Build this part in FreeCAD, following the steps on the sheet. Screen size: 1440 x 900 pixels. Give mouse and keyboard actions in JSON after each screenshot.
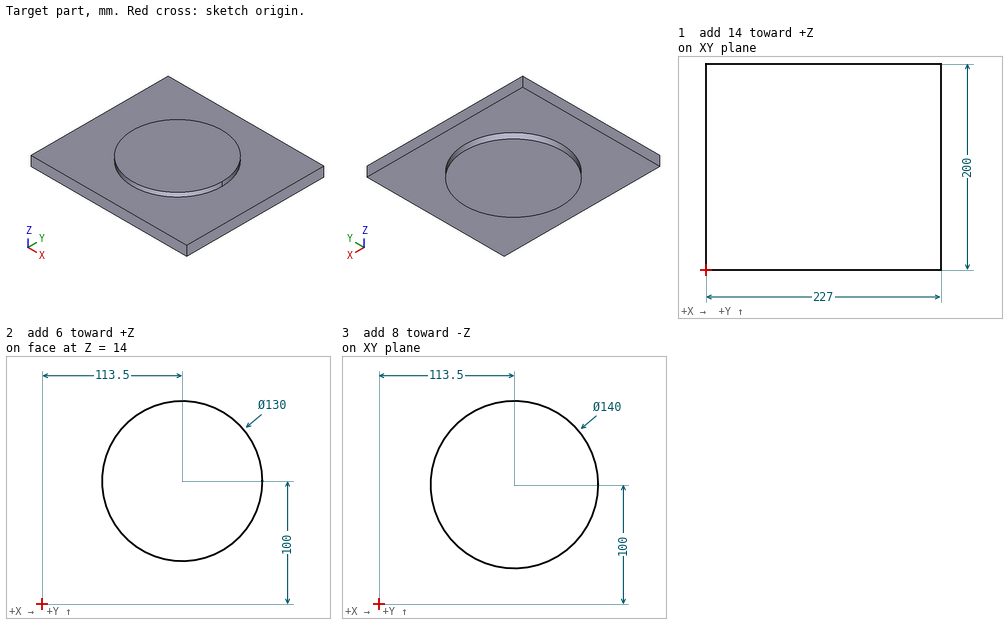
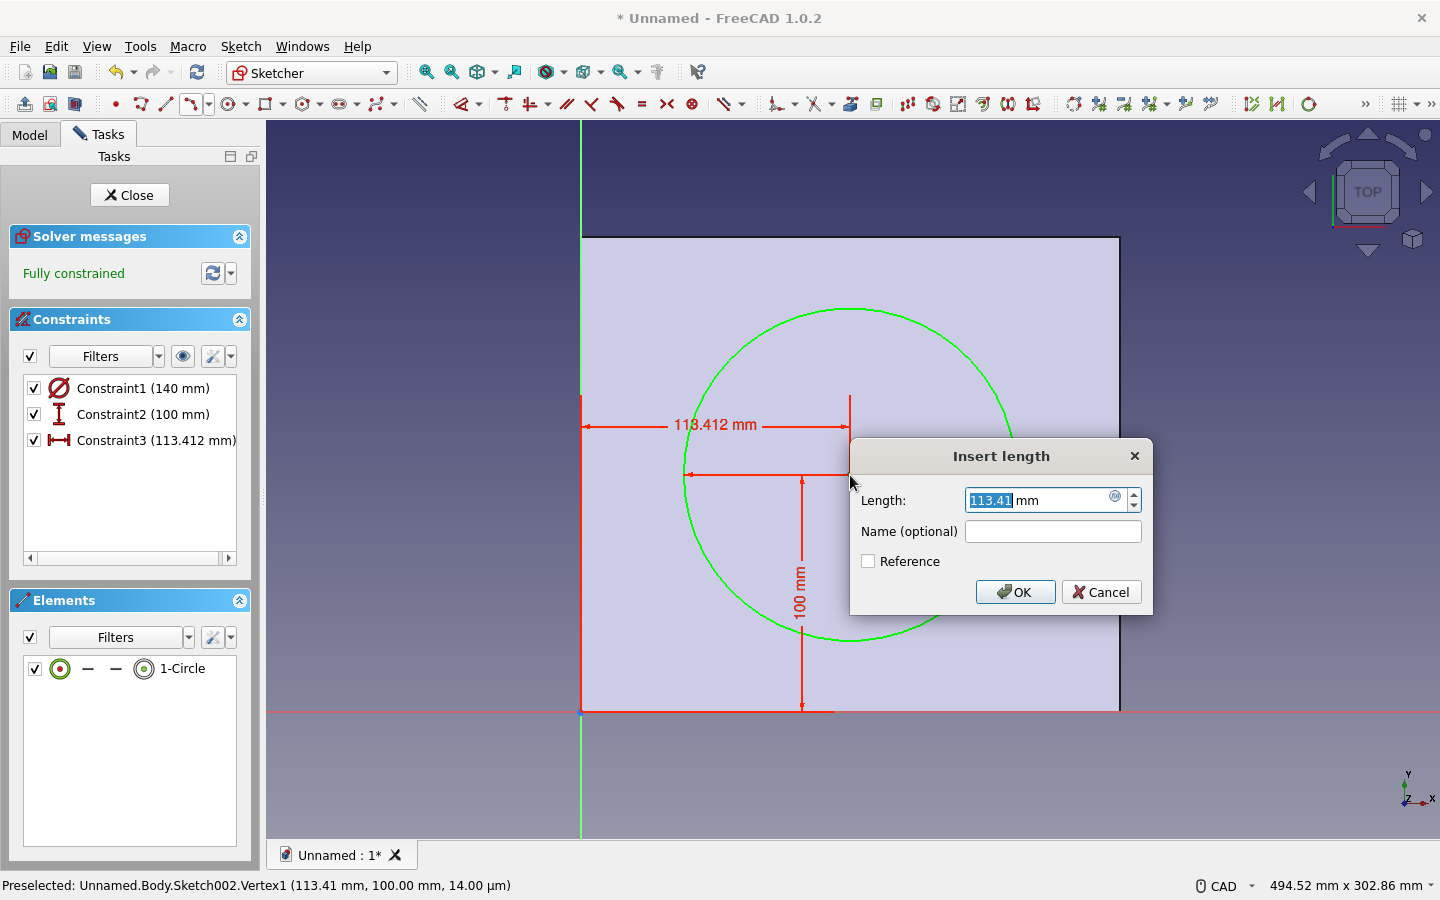
{"action": "type", "text": "113.5"}
{"action": "key", "text": "Return"}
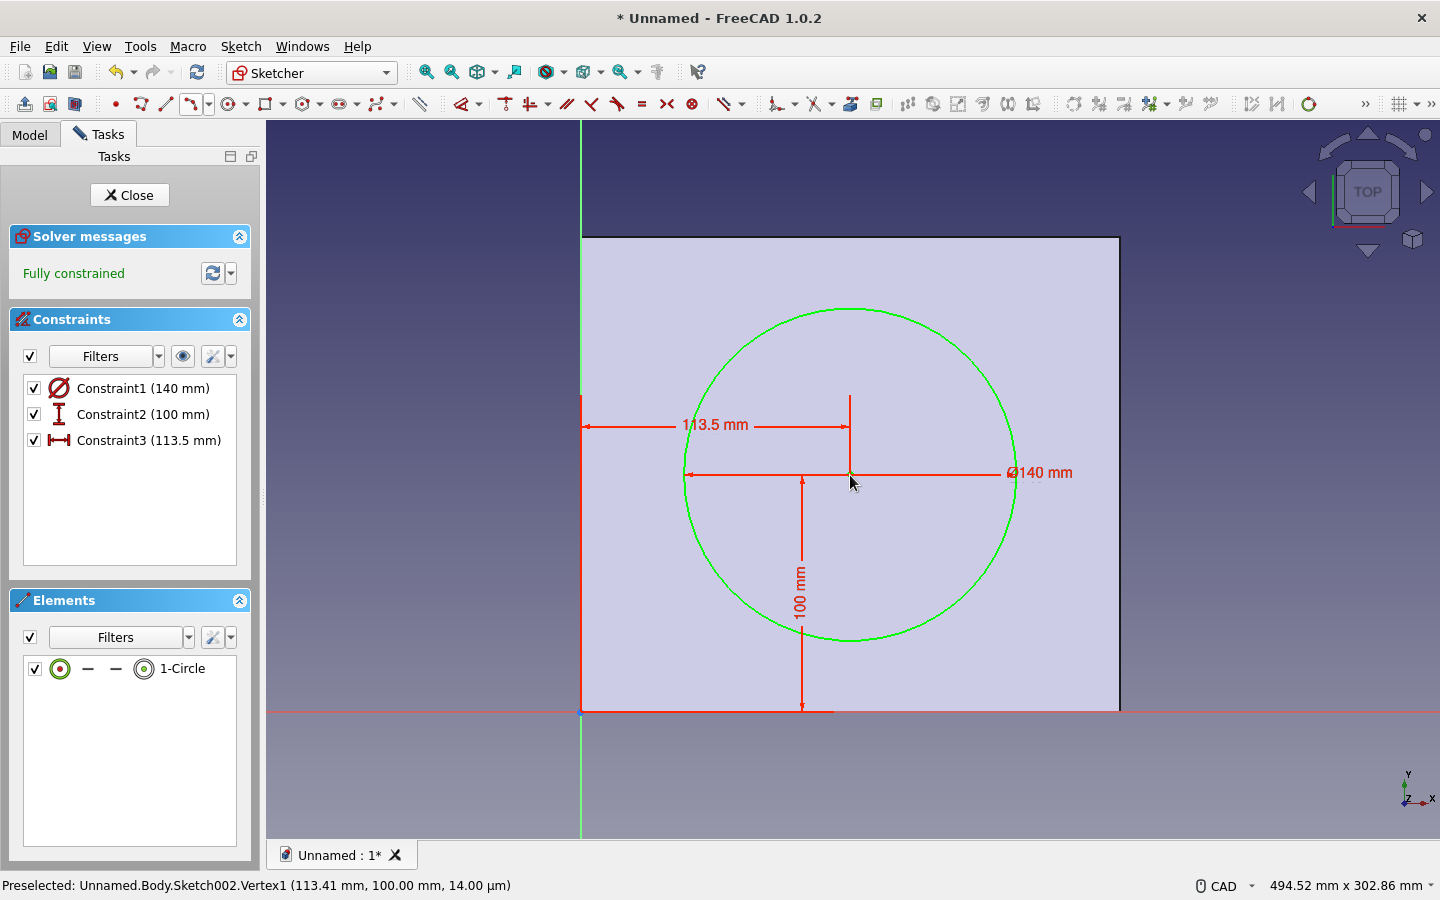
{"action": "left_click", "coordinate": [130, 195]}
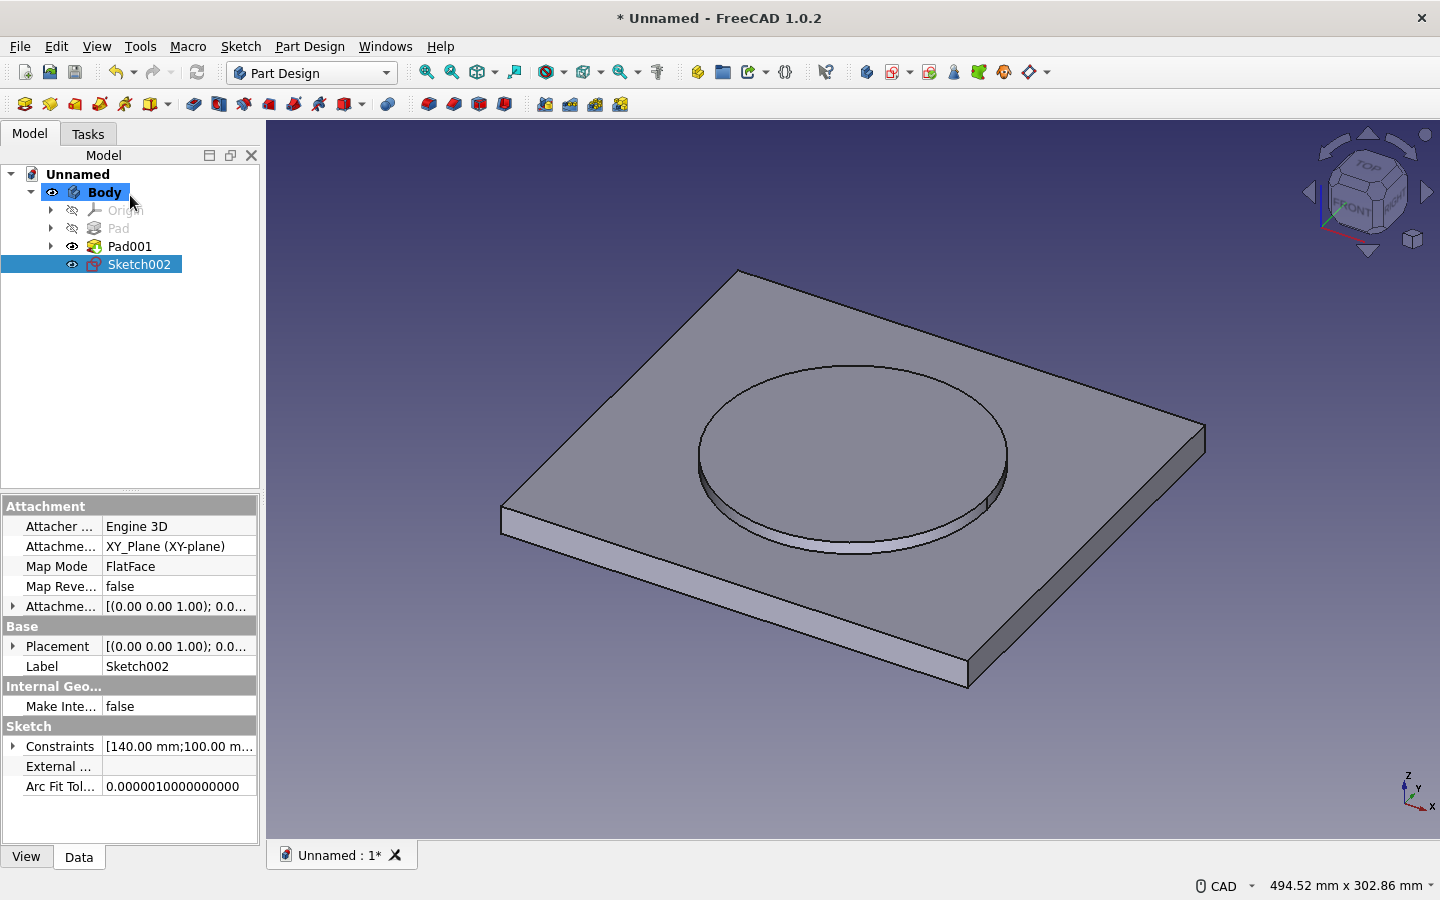
{"action": "left_click", "coordinate": [25, 104]}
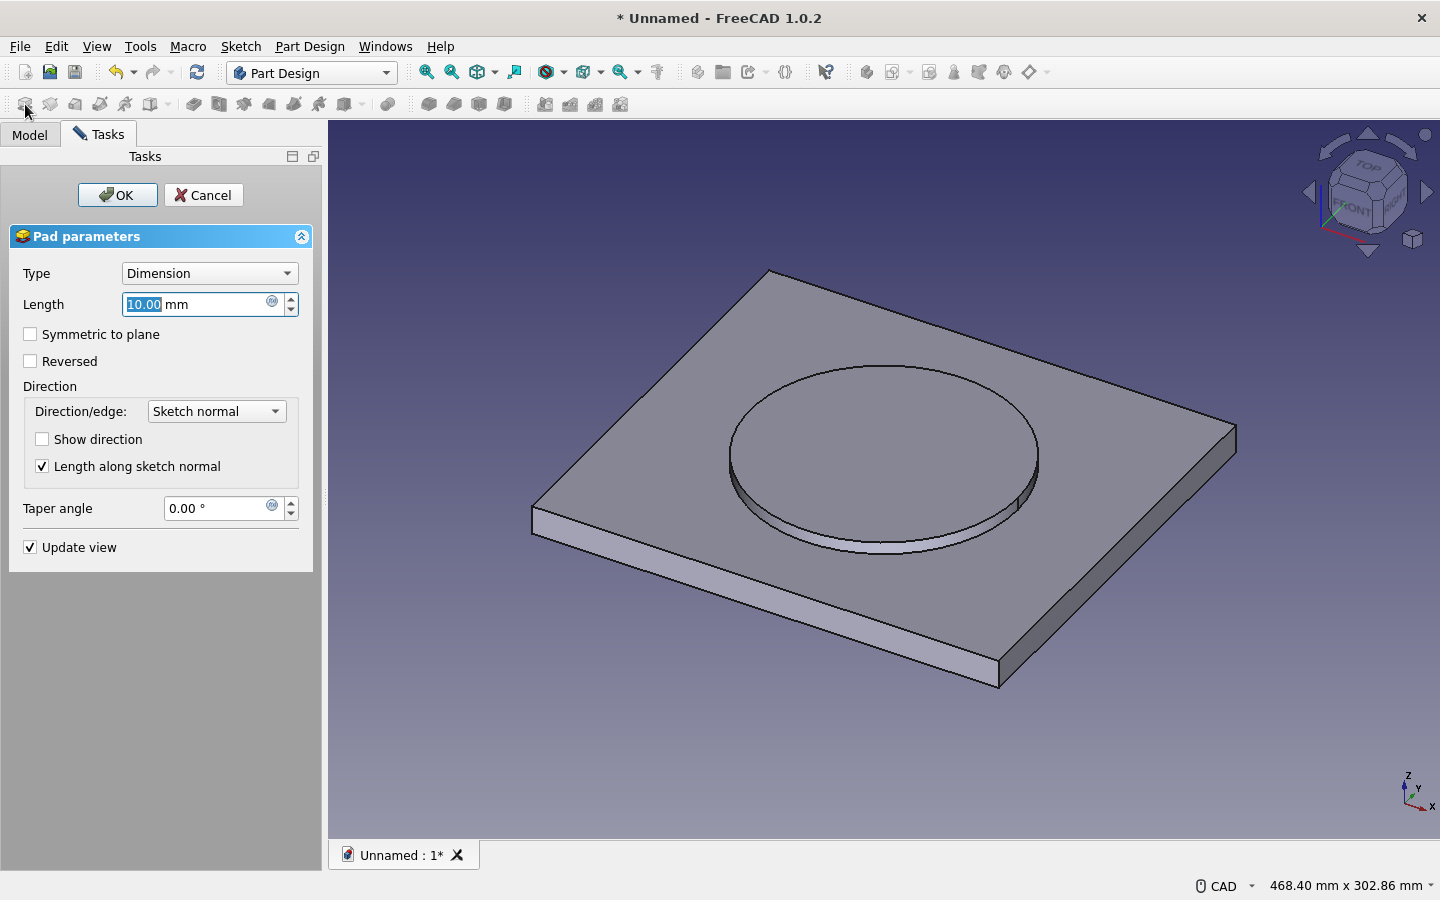
{"action": "type", "text": "8"}
{"action": "key", "text": "Tab"}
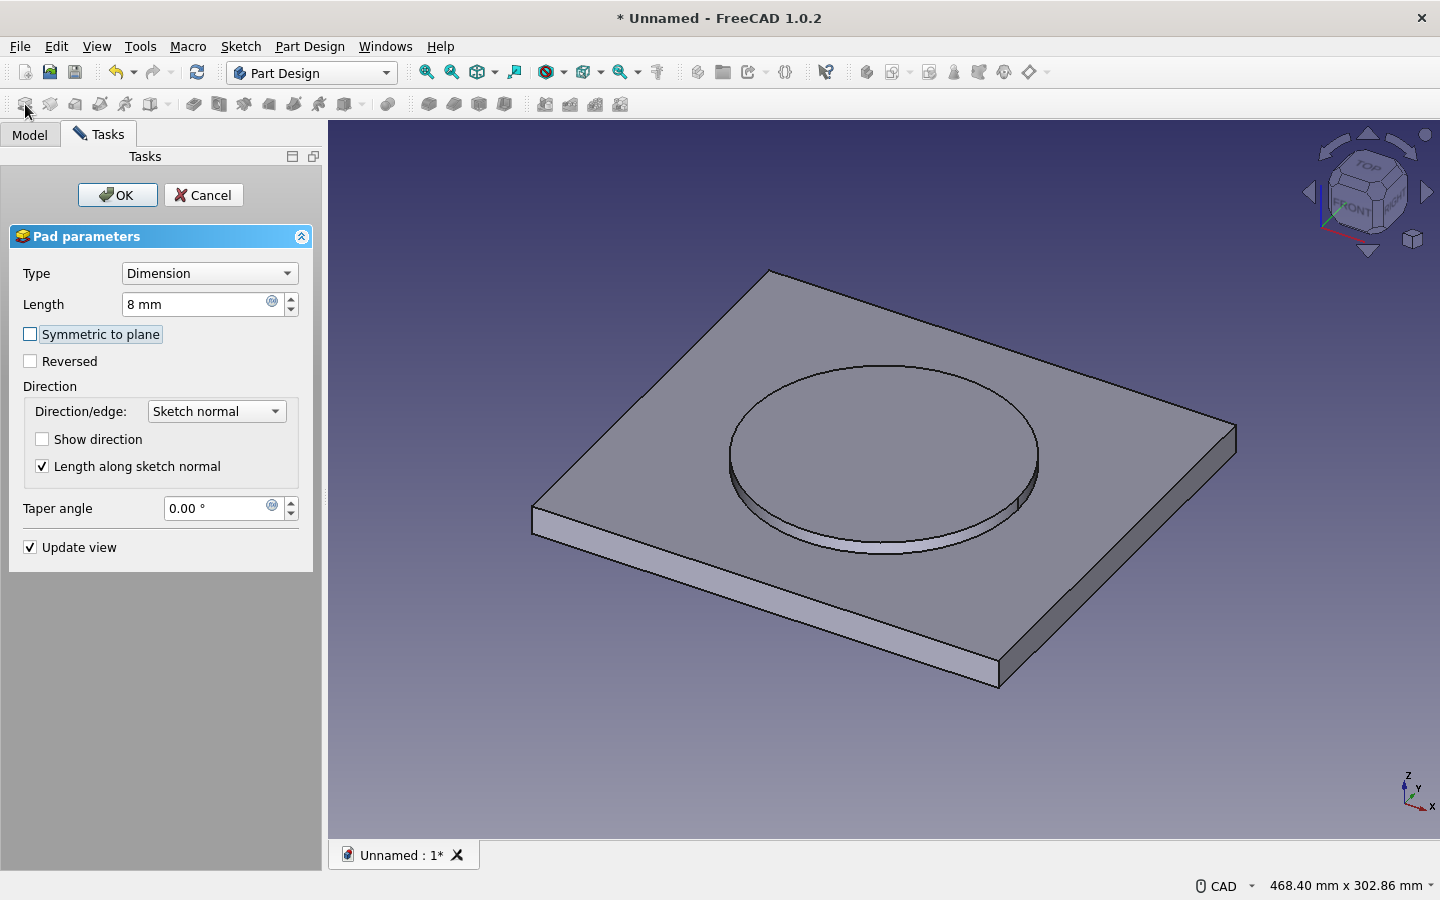
{"action": "left_click", "coordinate": [31, 361]}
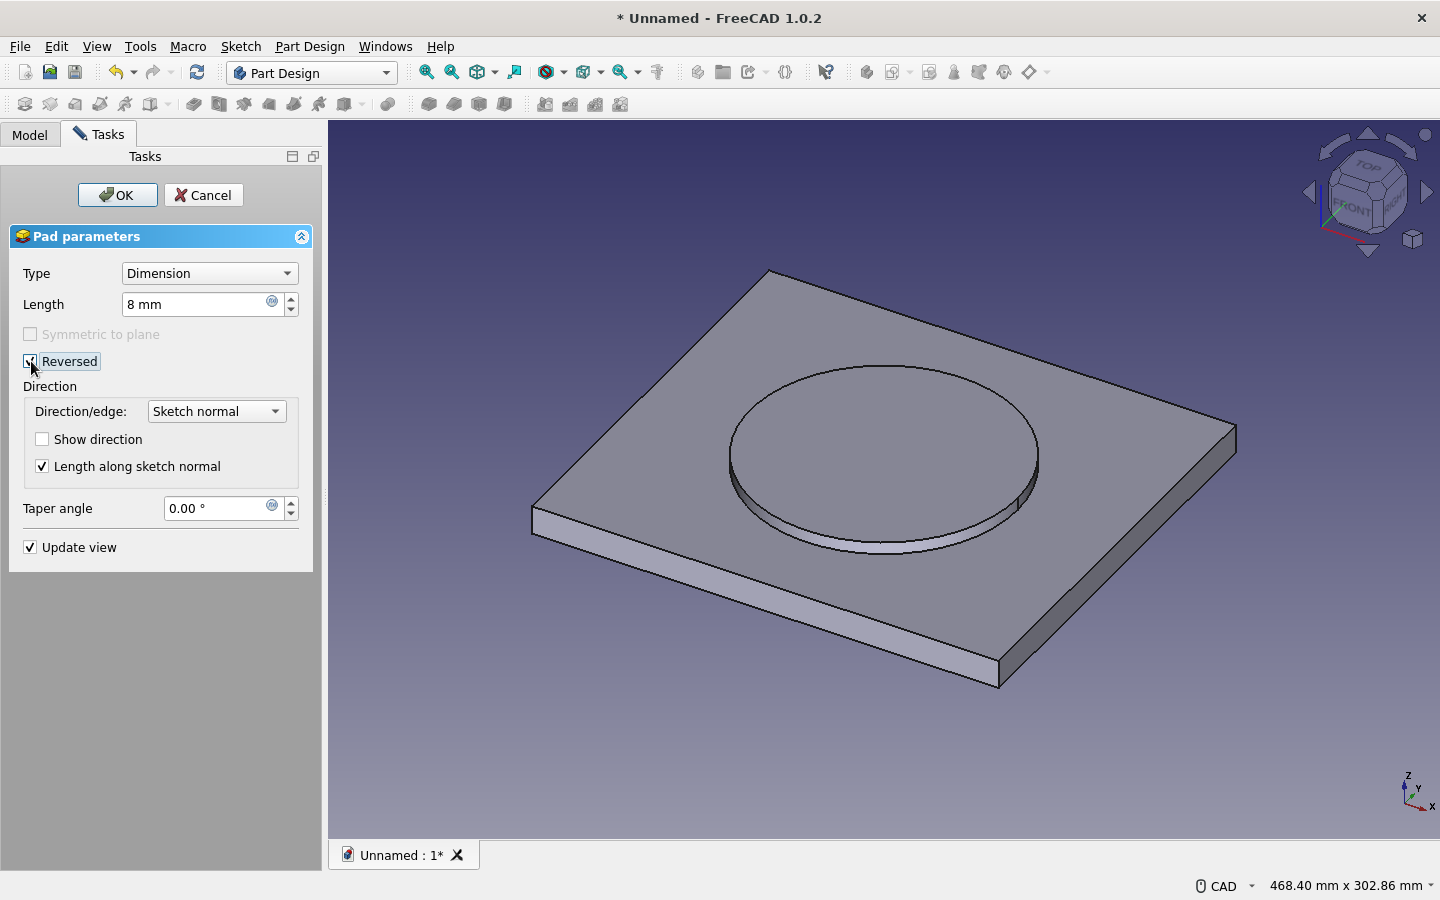
{"action": "left_click", "coordinate": [118, 195]}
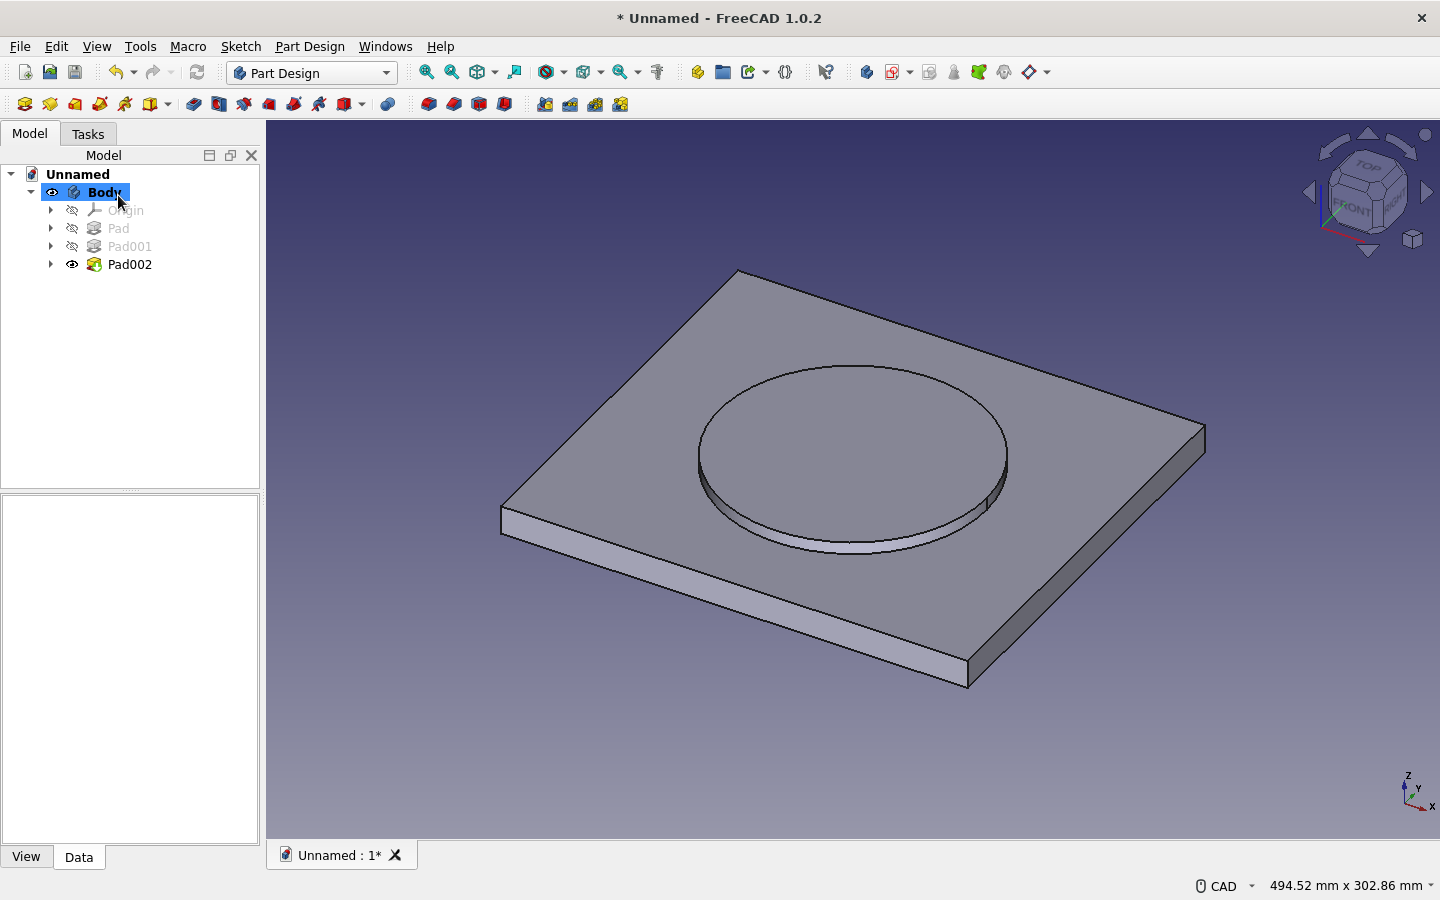
{"action": "key", "text": "0"}